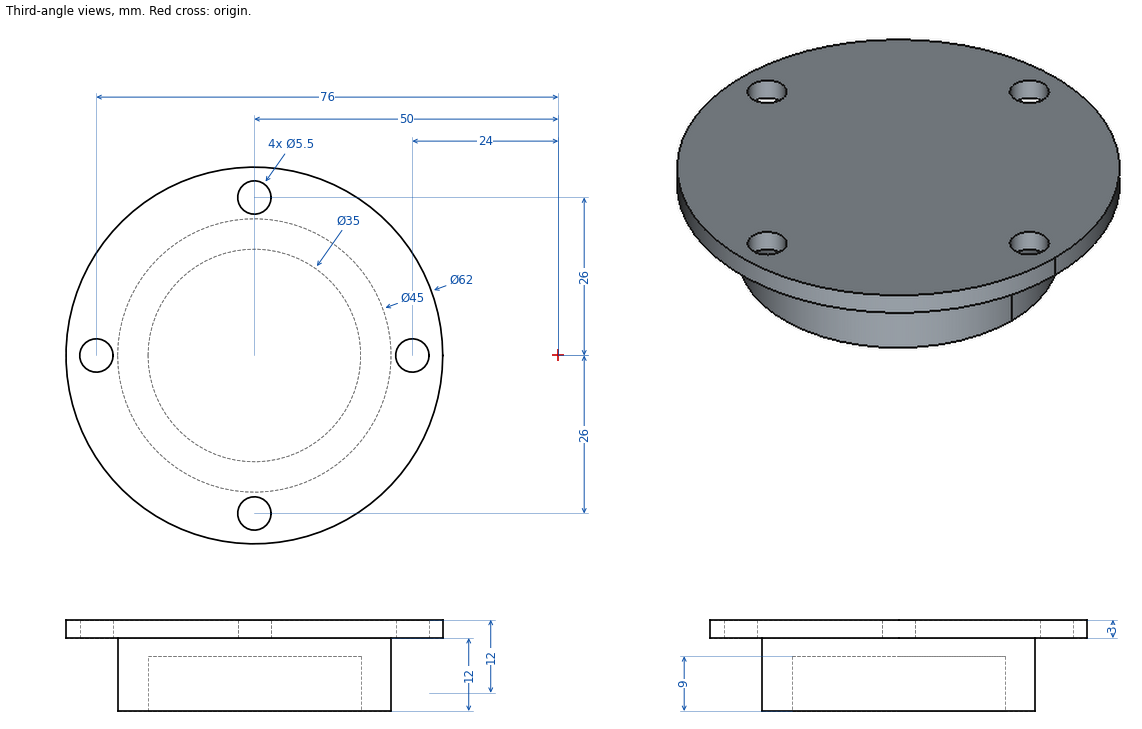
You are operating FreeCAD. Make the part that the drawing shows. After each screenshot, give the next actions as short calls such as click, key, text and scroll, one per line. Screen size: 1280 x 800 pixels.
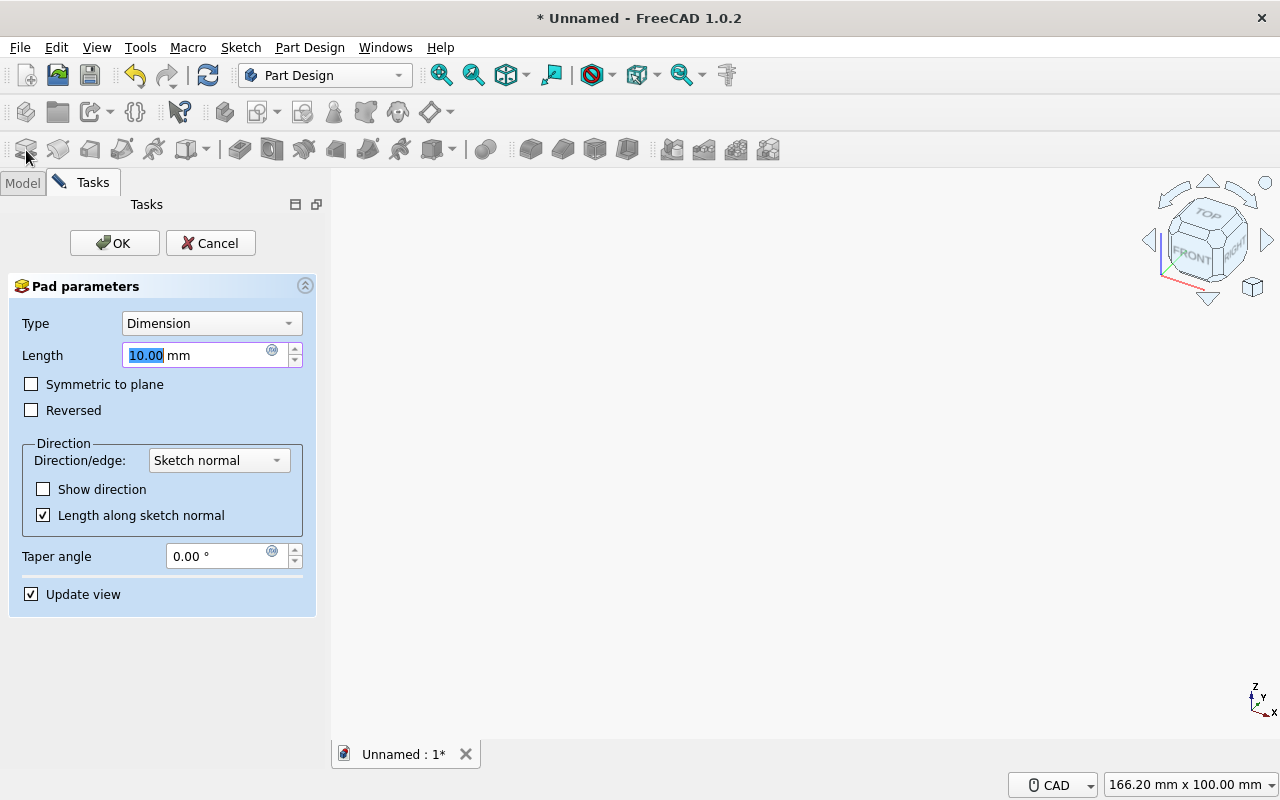
text(3)
key(Tab)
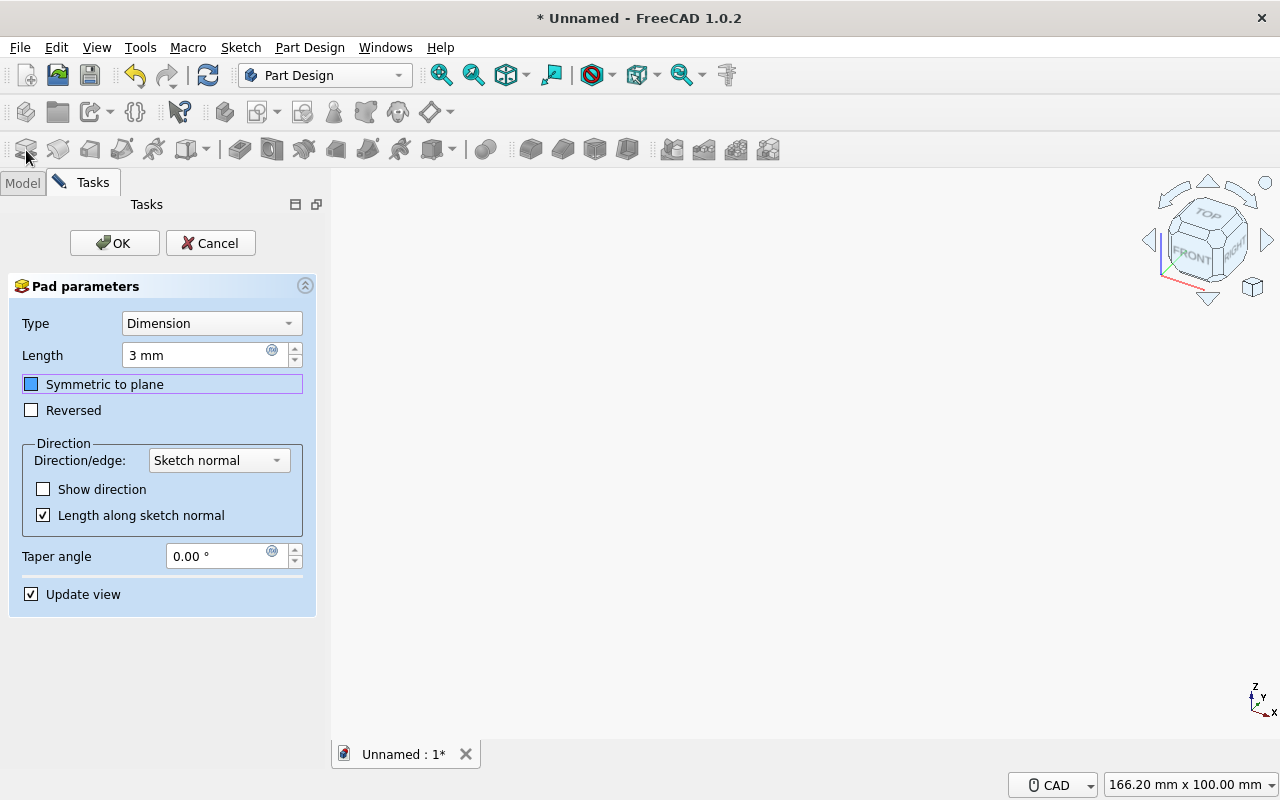
click(115, 243)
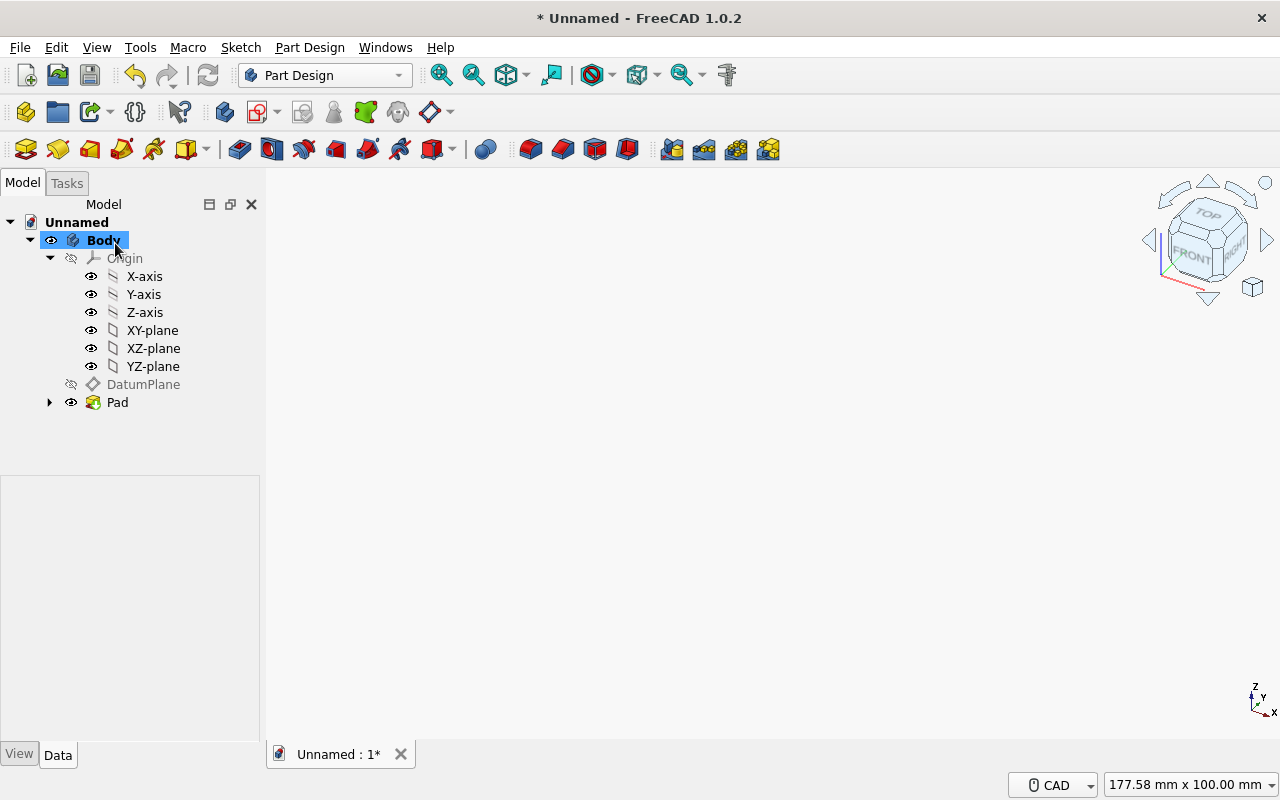
click(442, 76)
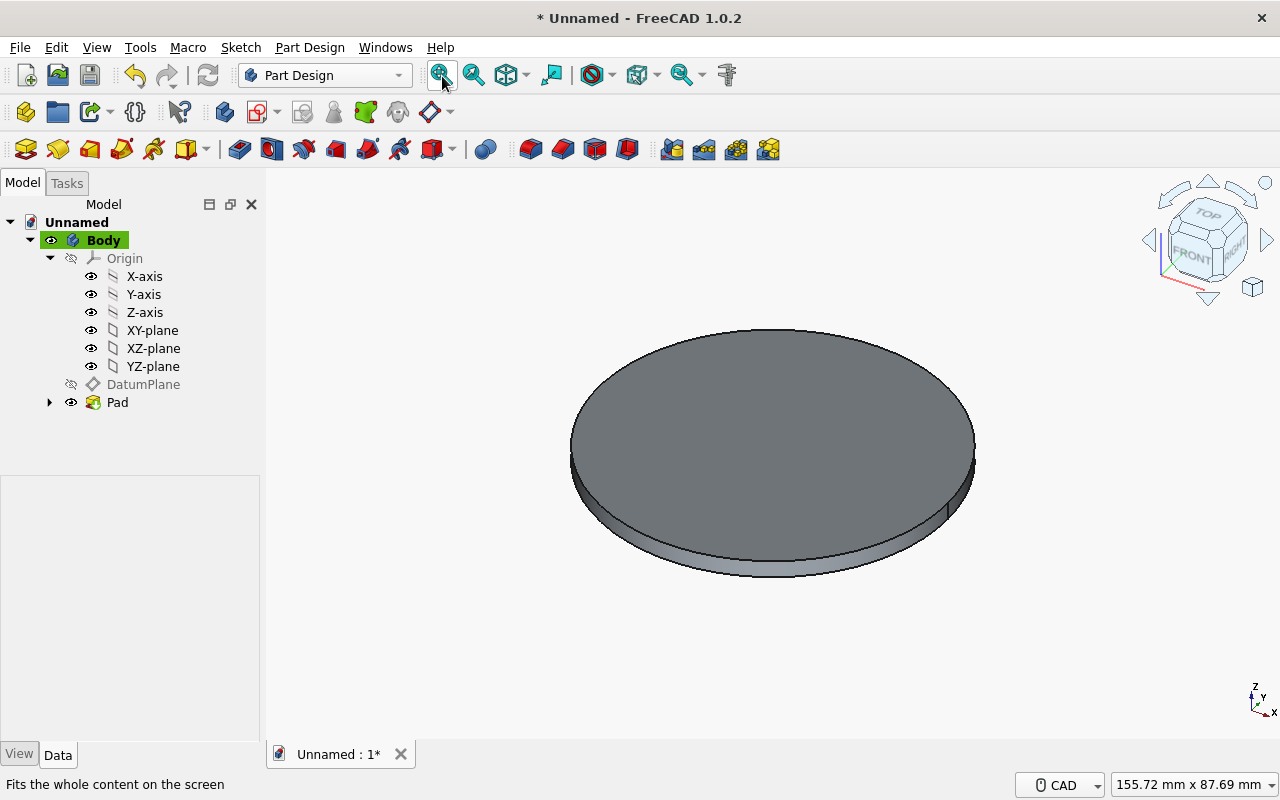
key(5)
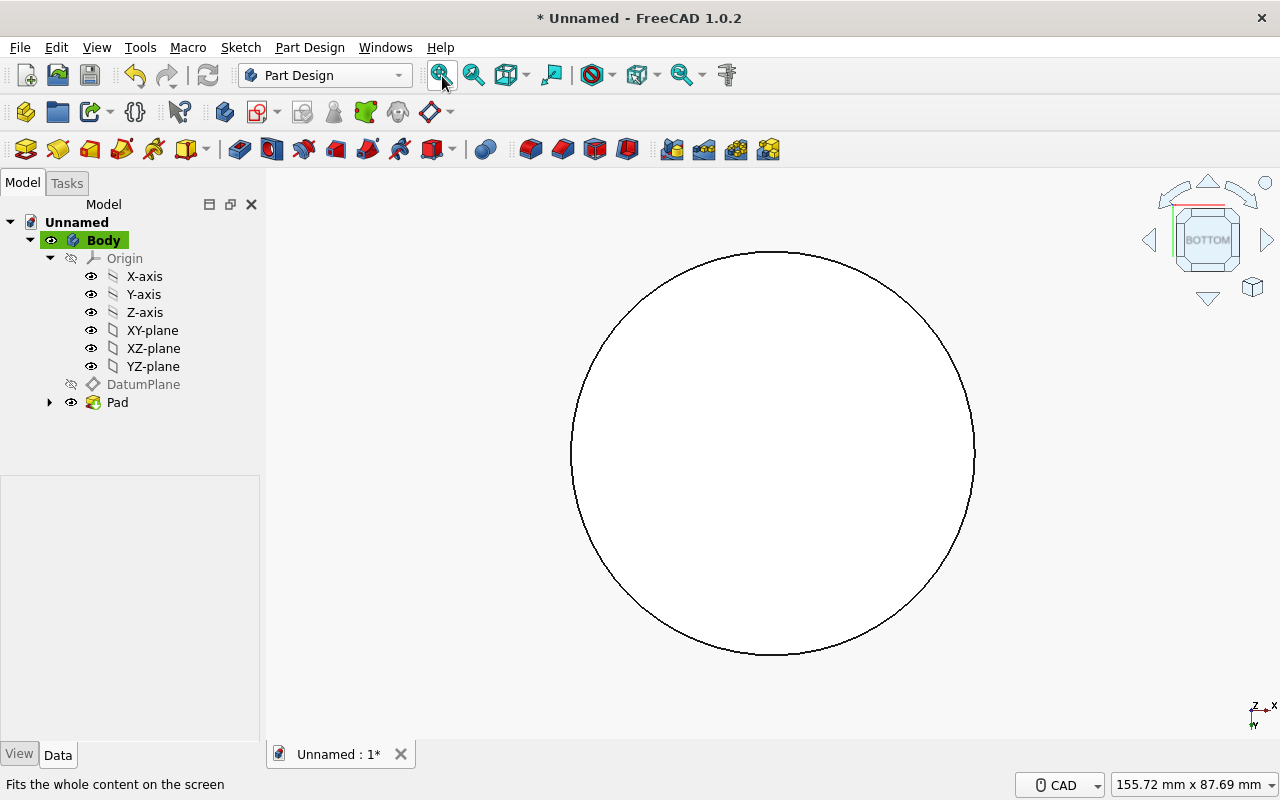
click(773, 452)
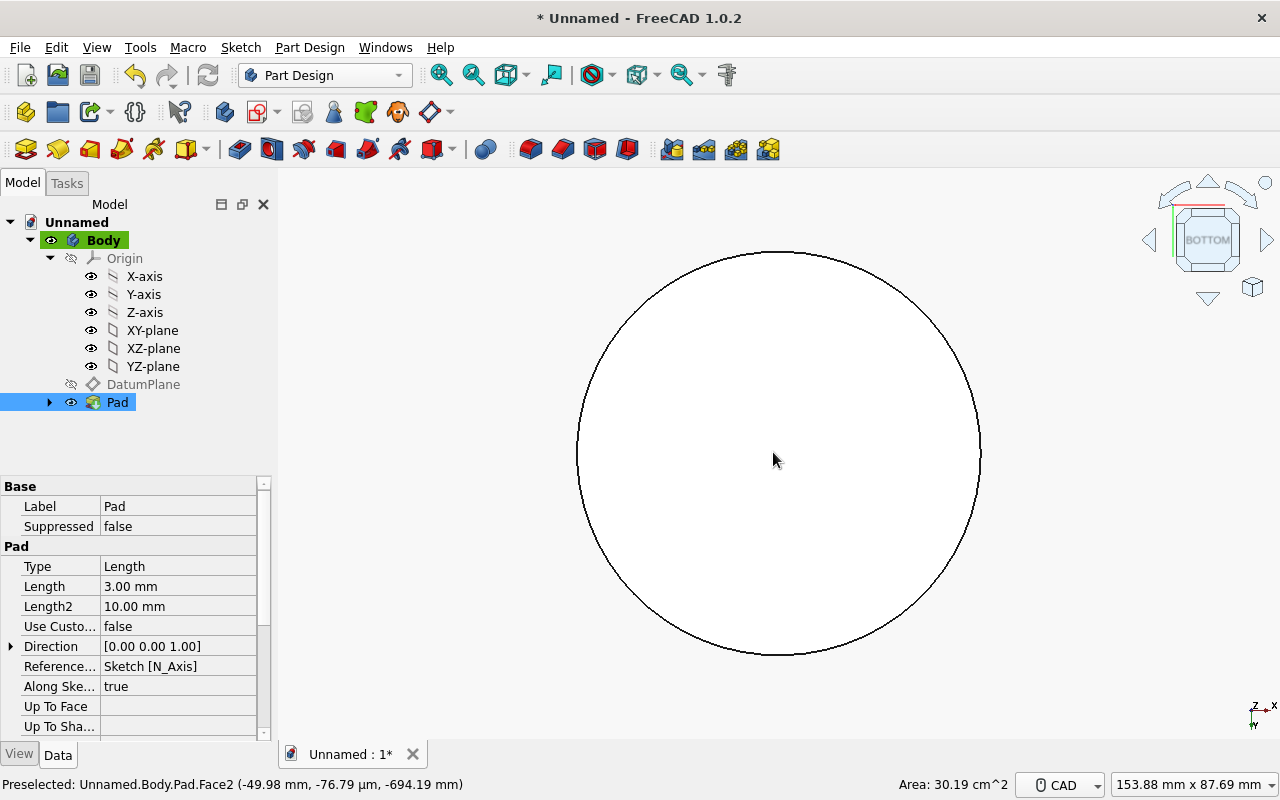
click(258, 112)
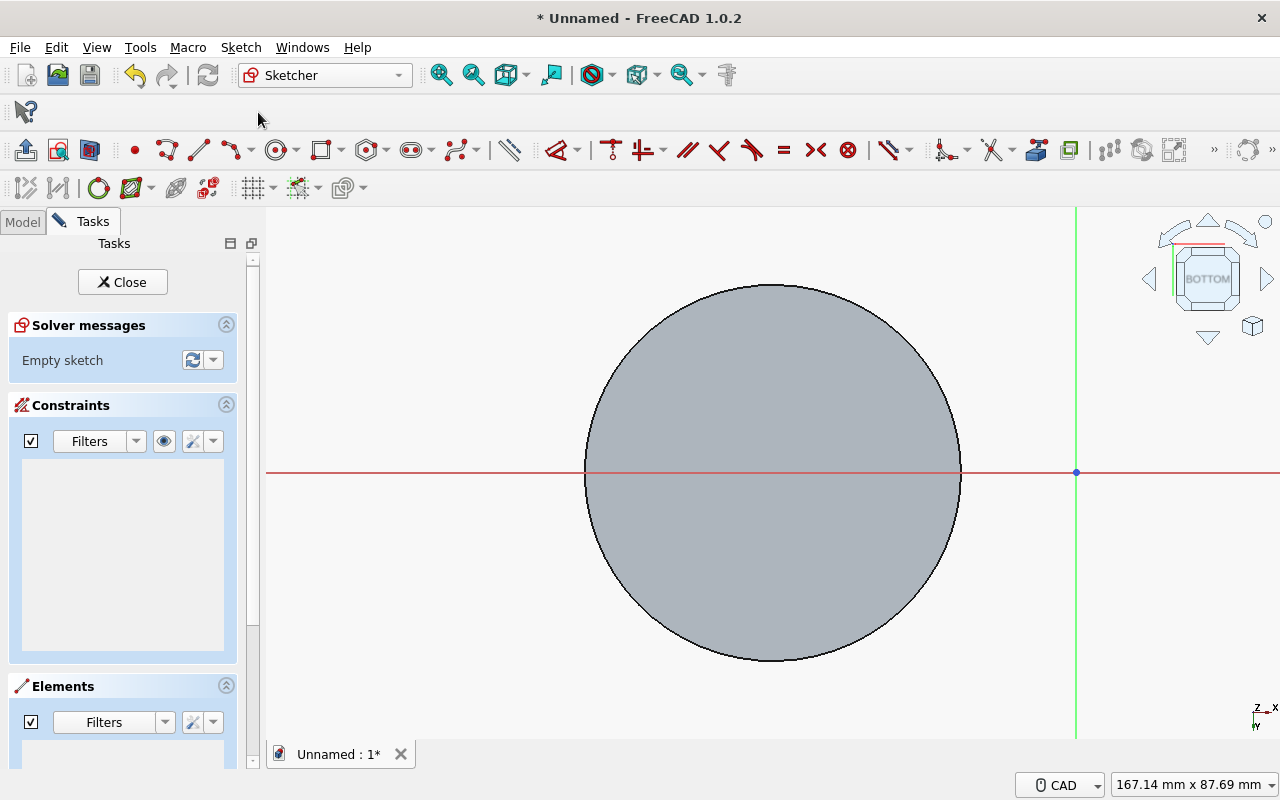
click(276, 150)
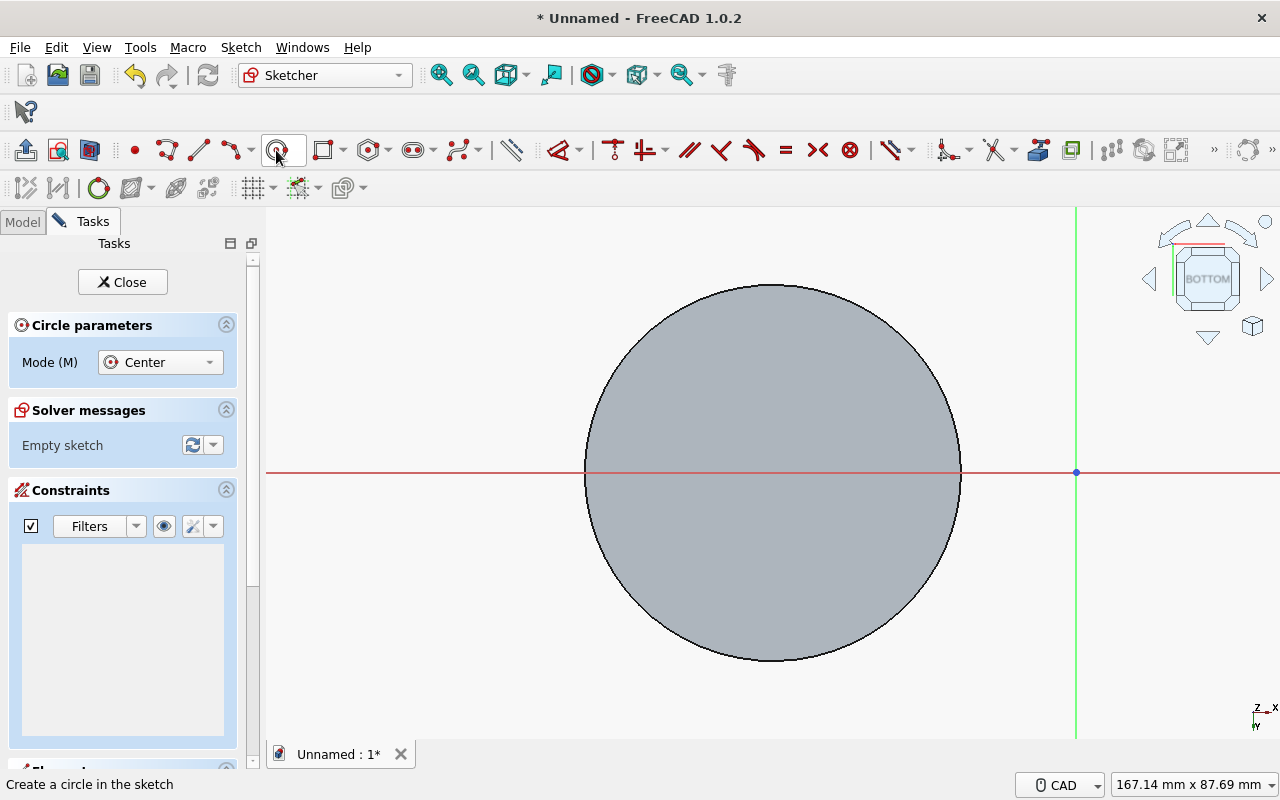
click(773, 473)
move(869, 376)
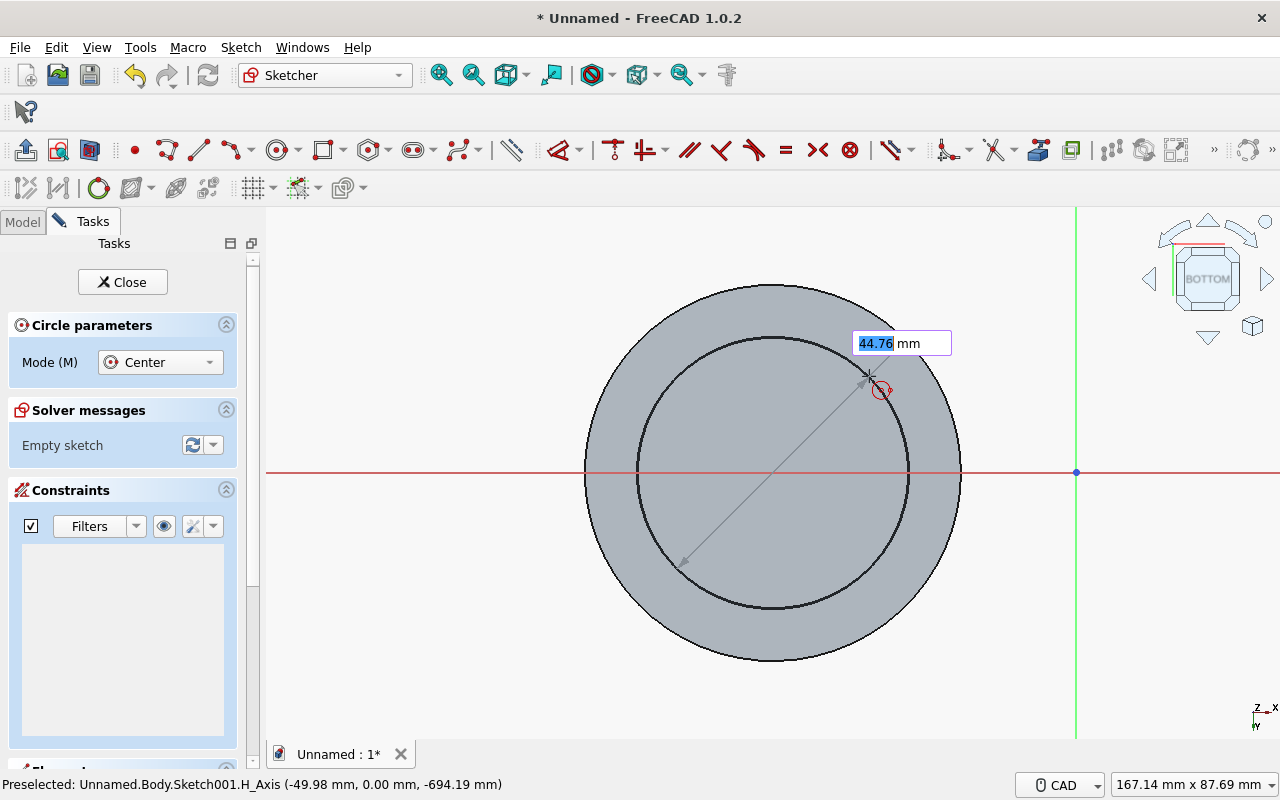
text(45)
key(Return)
key(Escape)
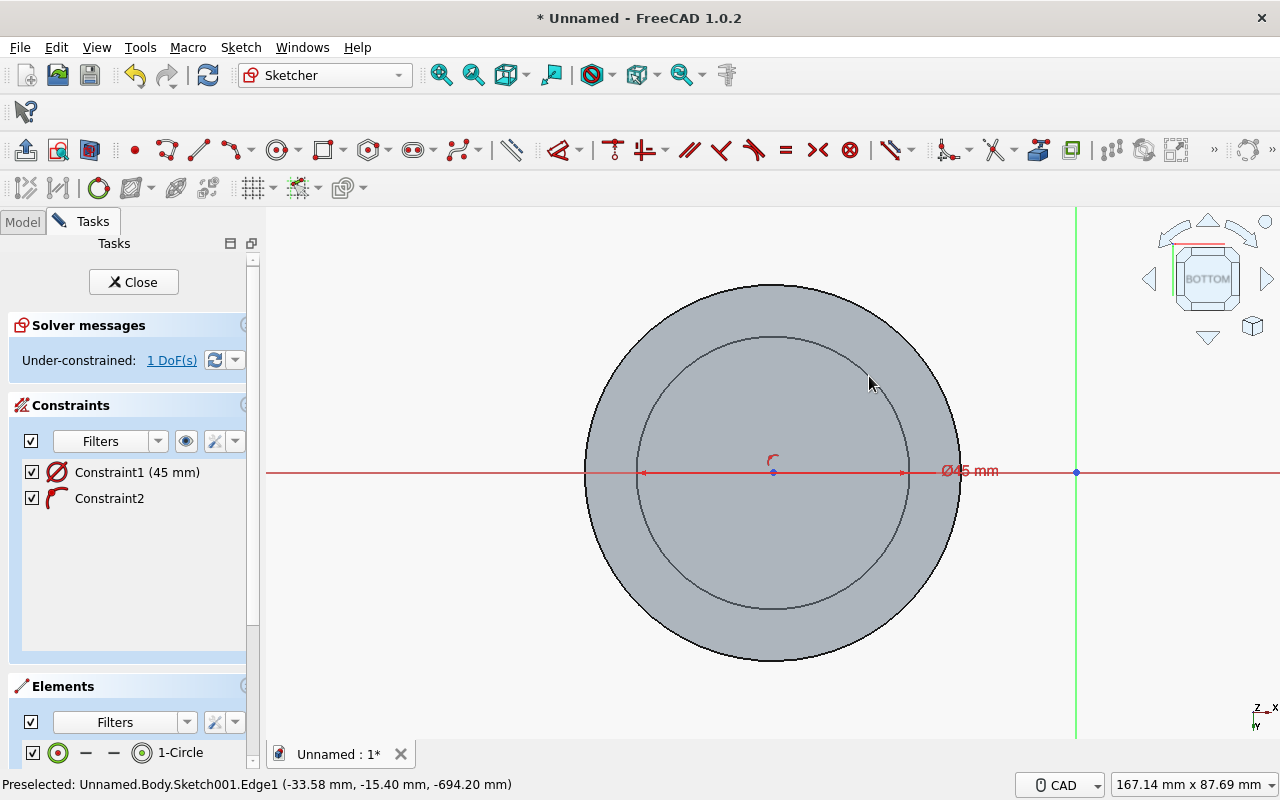
click(558, 150)